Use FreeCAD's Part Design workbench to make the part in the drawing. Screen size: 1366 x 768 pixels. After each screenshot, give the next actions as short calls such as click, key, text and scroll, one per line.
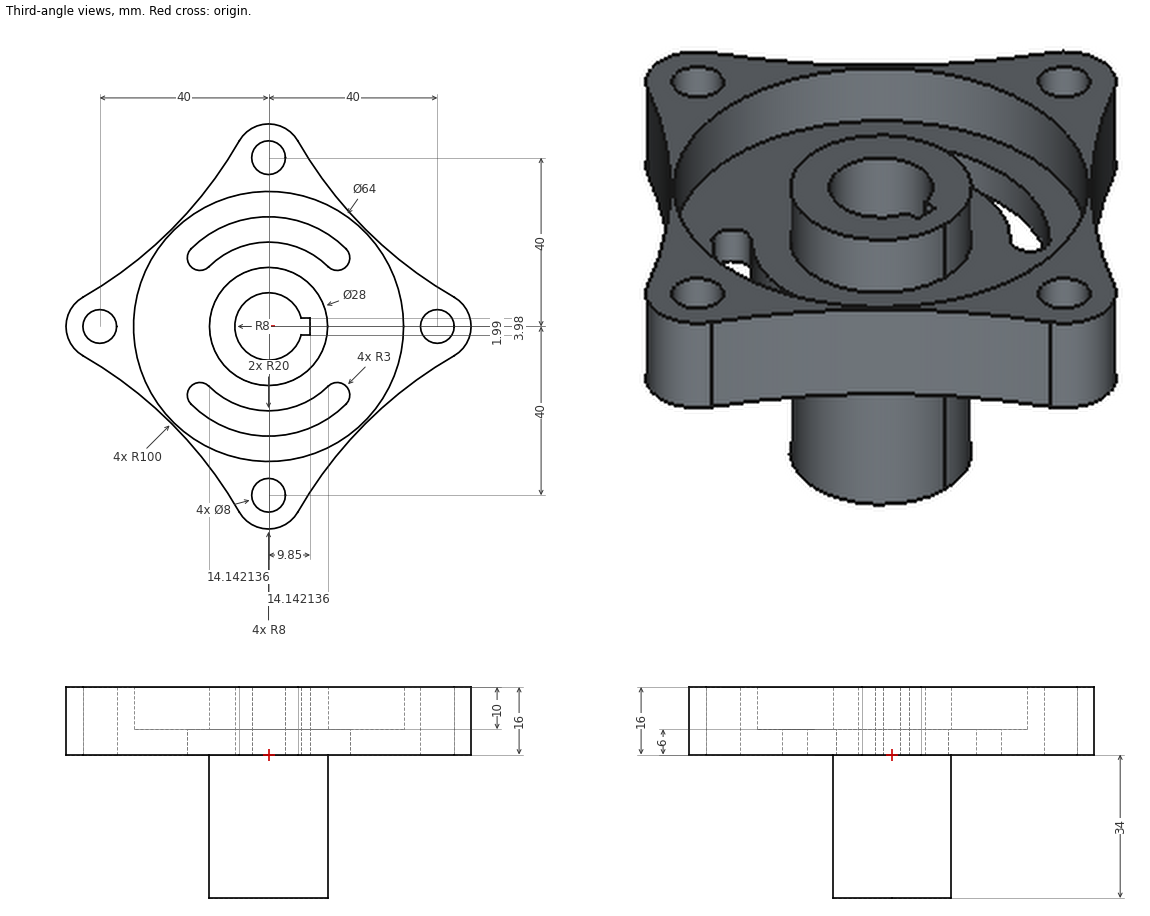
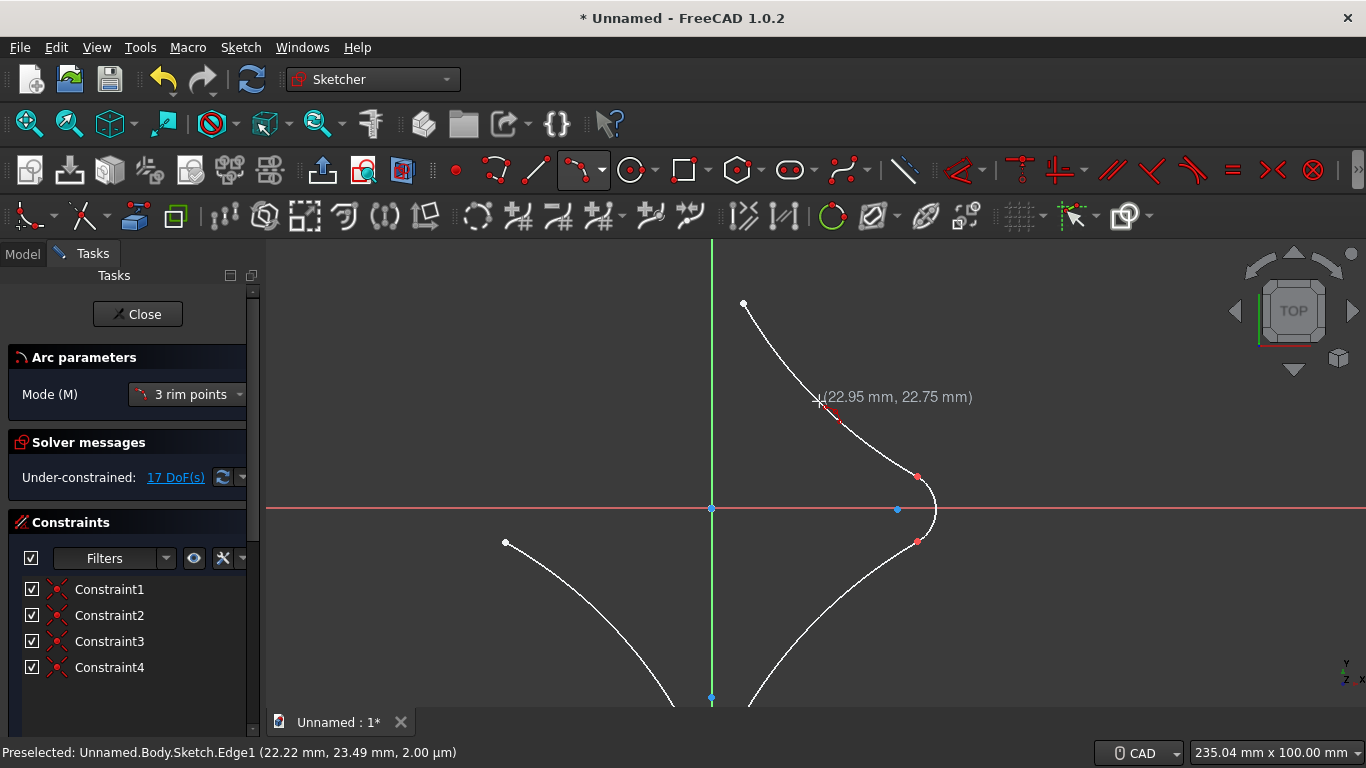
click(744, 304)
click(679, 303)
click(727, 287)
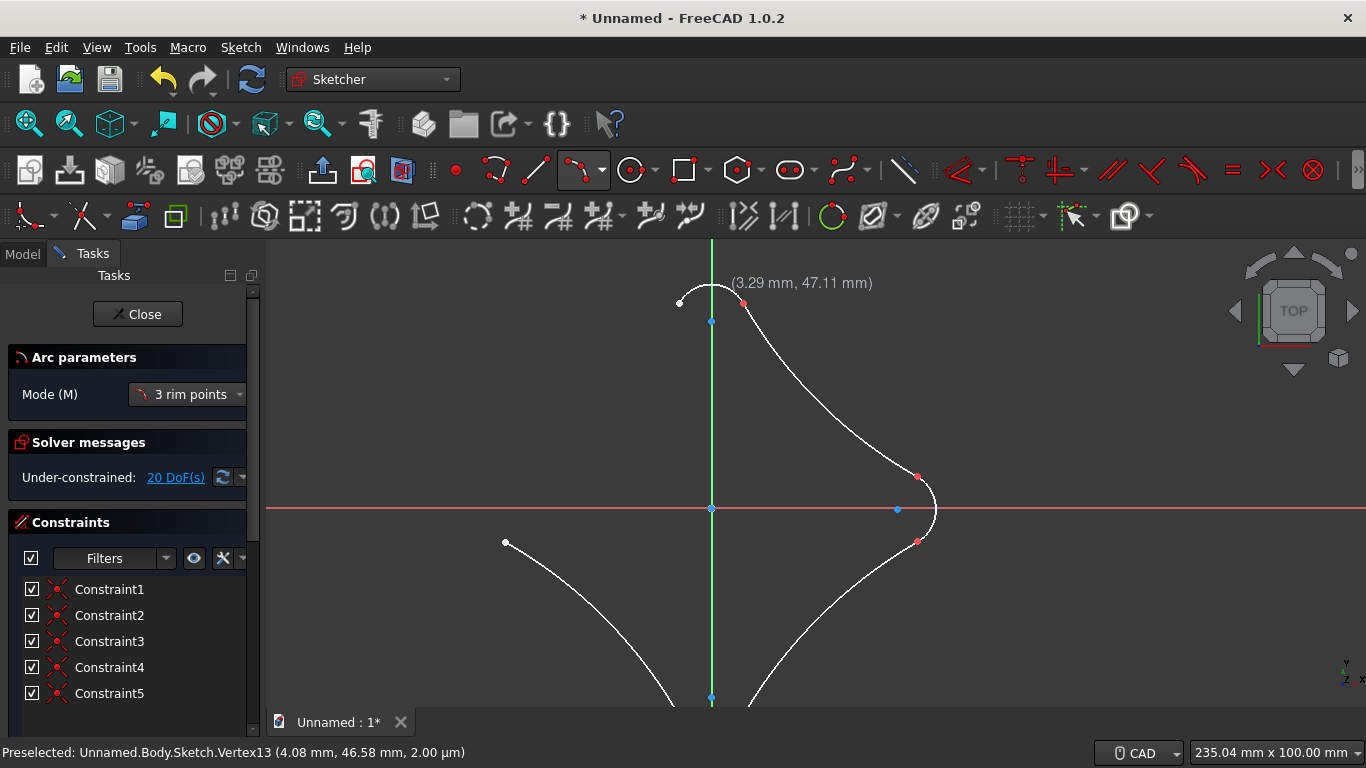
click(679, 304)
click(506, 476)
click(604, 401)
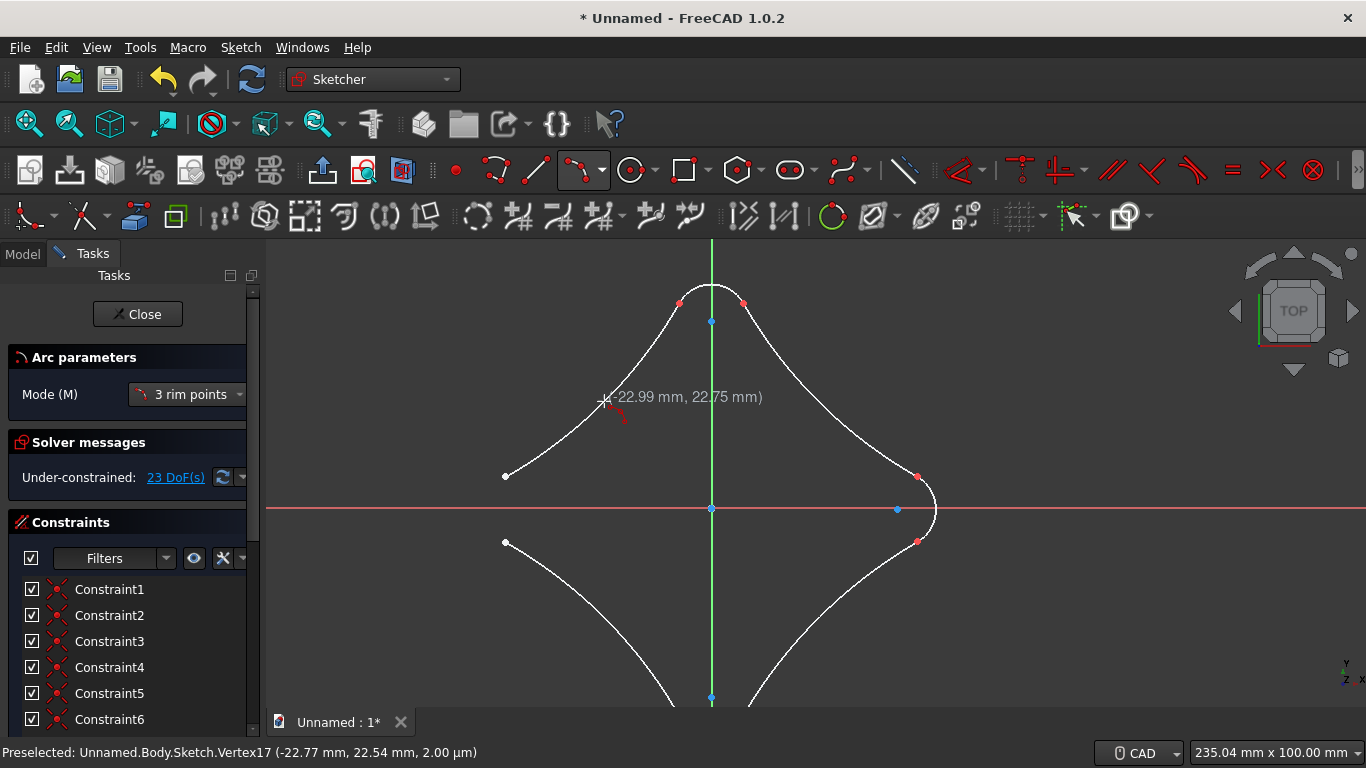
click(506, 477)
click(506, 543)
click(490, 493)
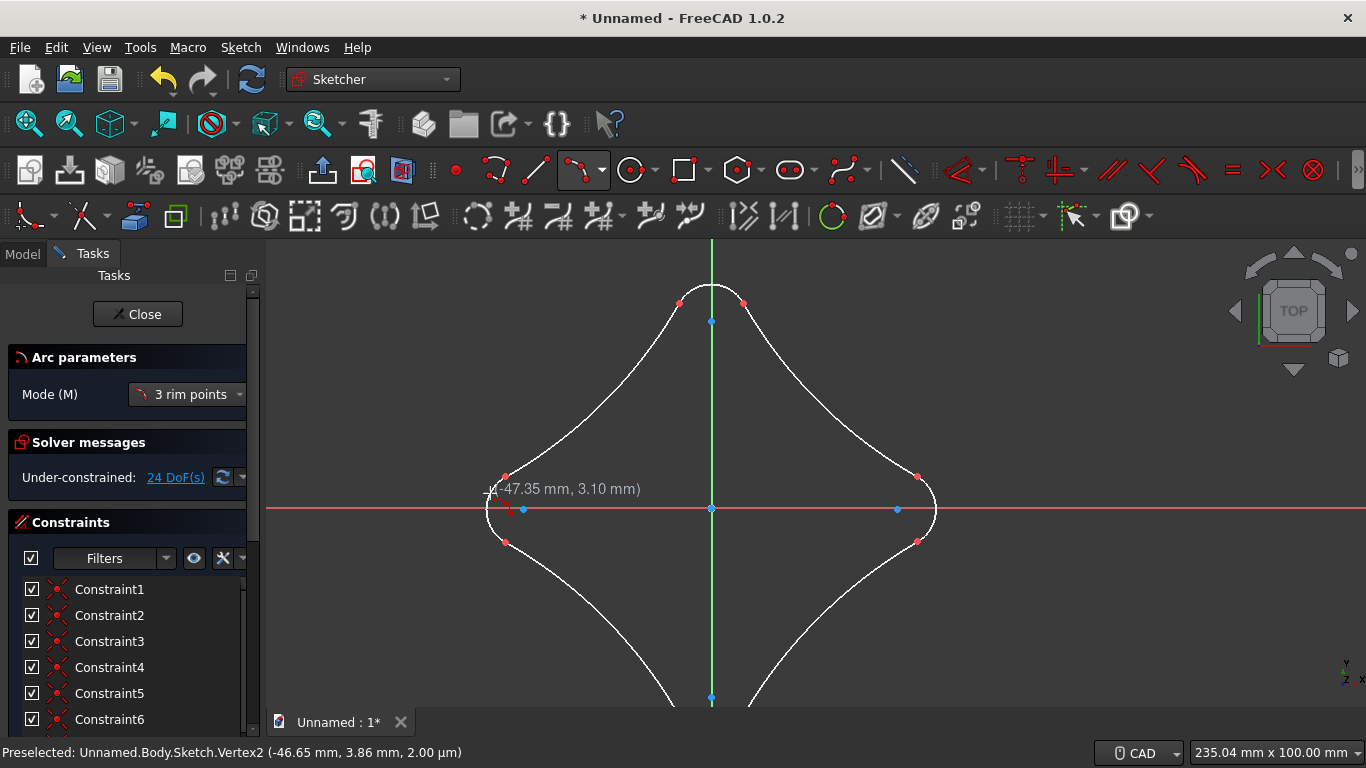
key(g)
key(c)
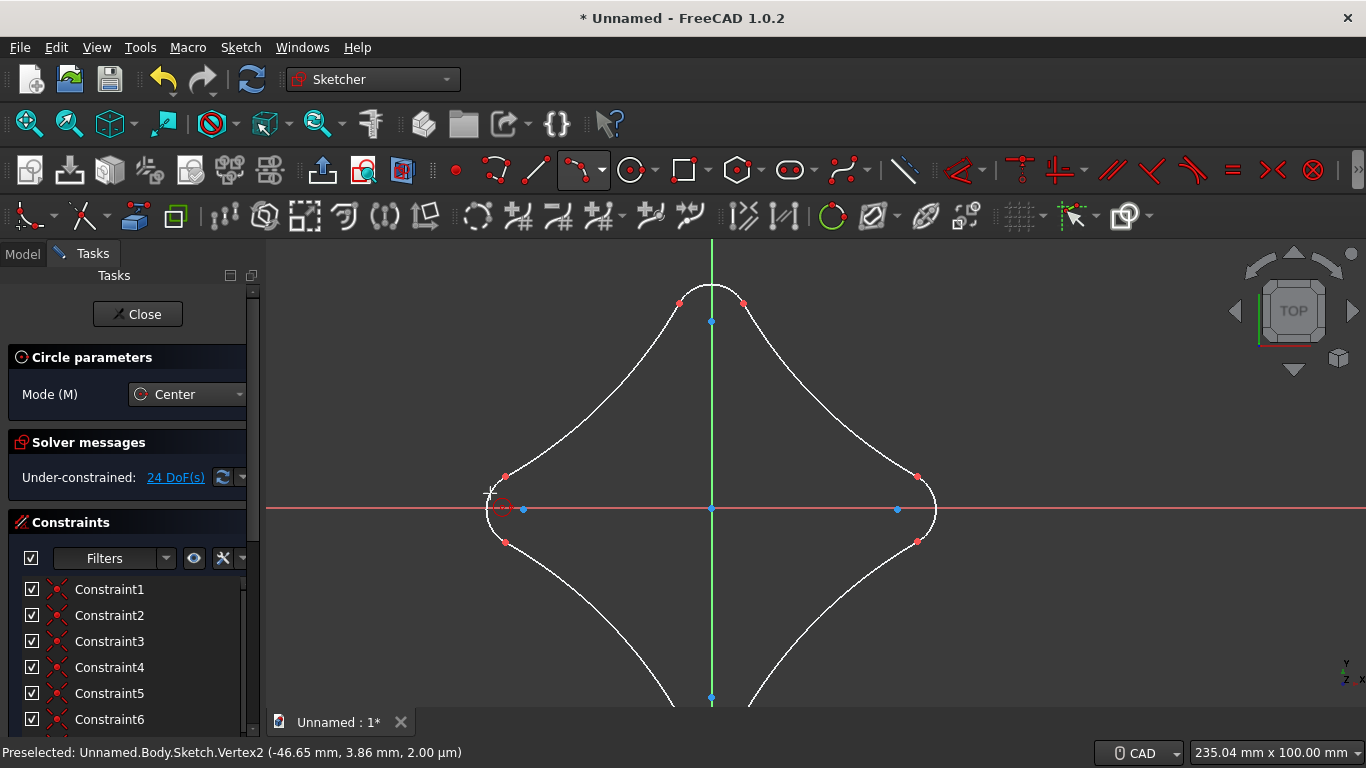
scroll(821, 401, down, 2)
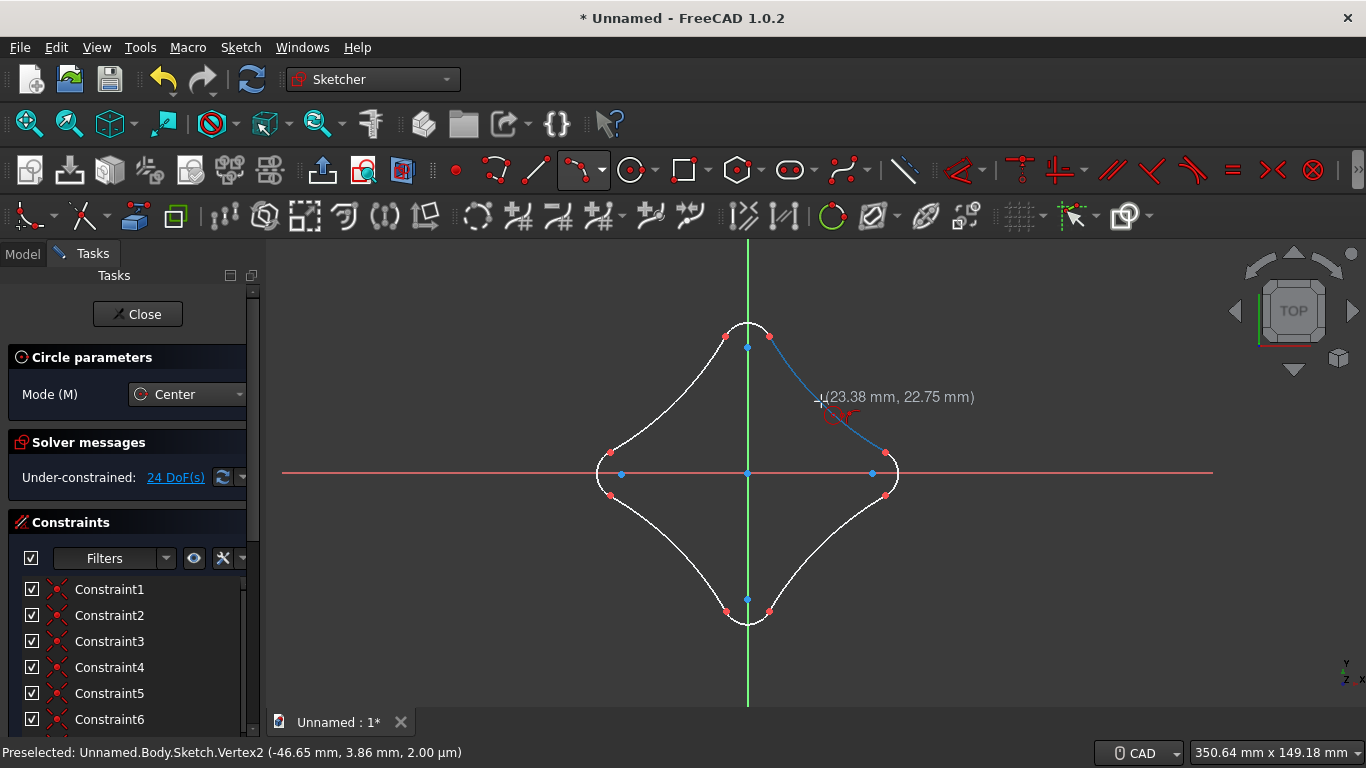
scroll(748, 599, up, 3)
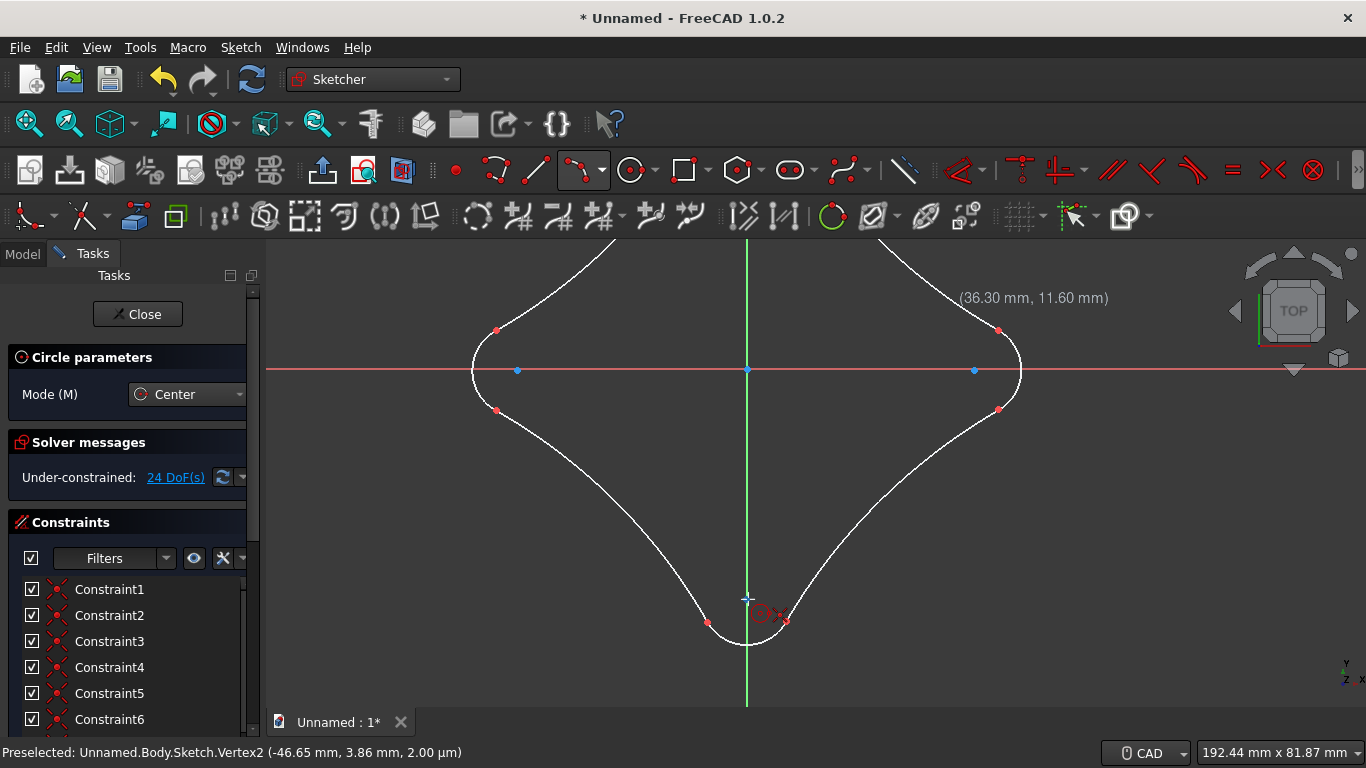
click(747, 598)
move(763, 582)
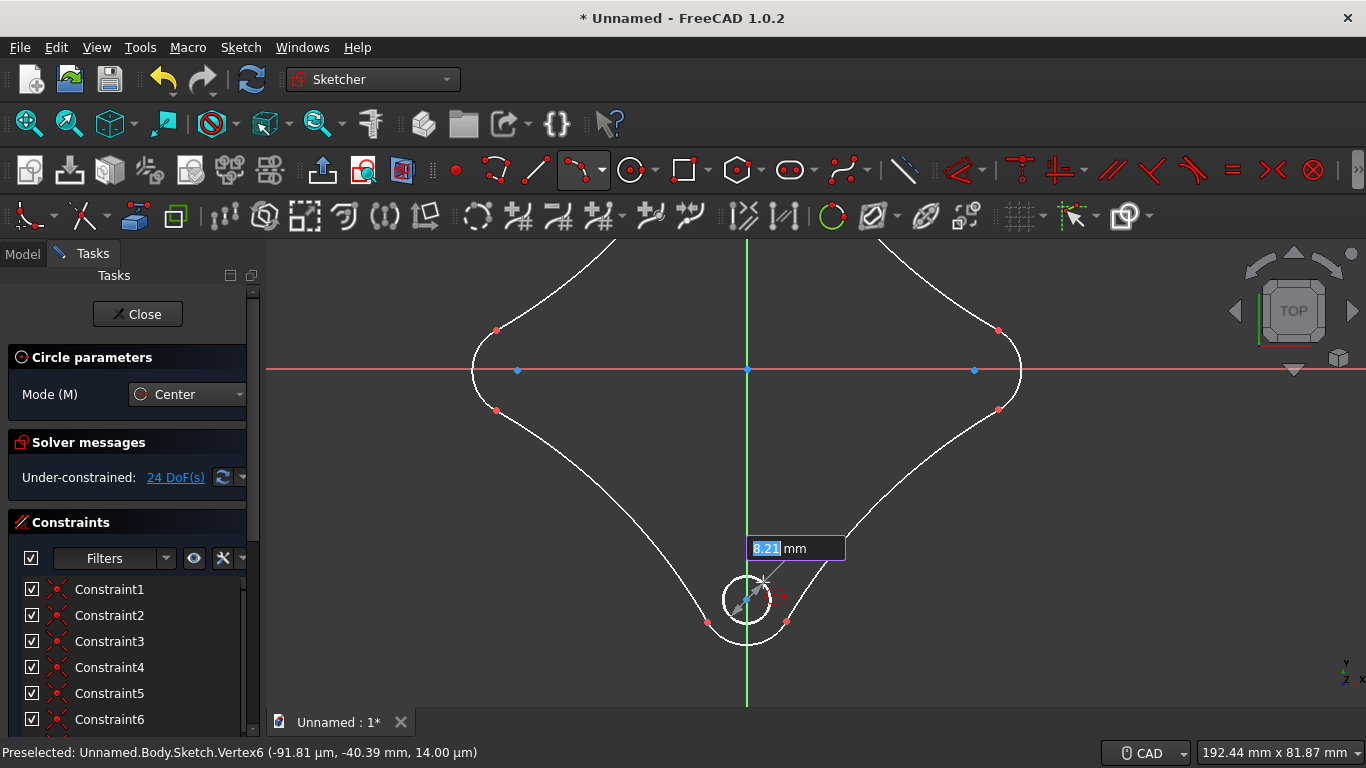
text(8)
key(Return)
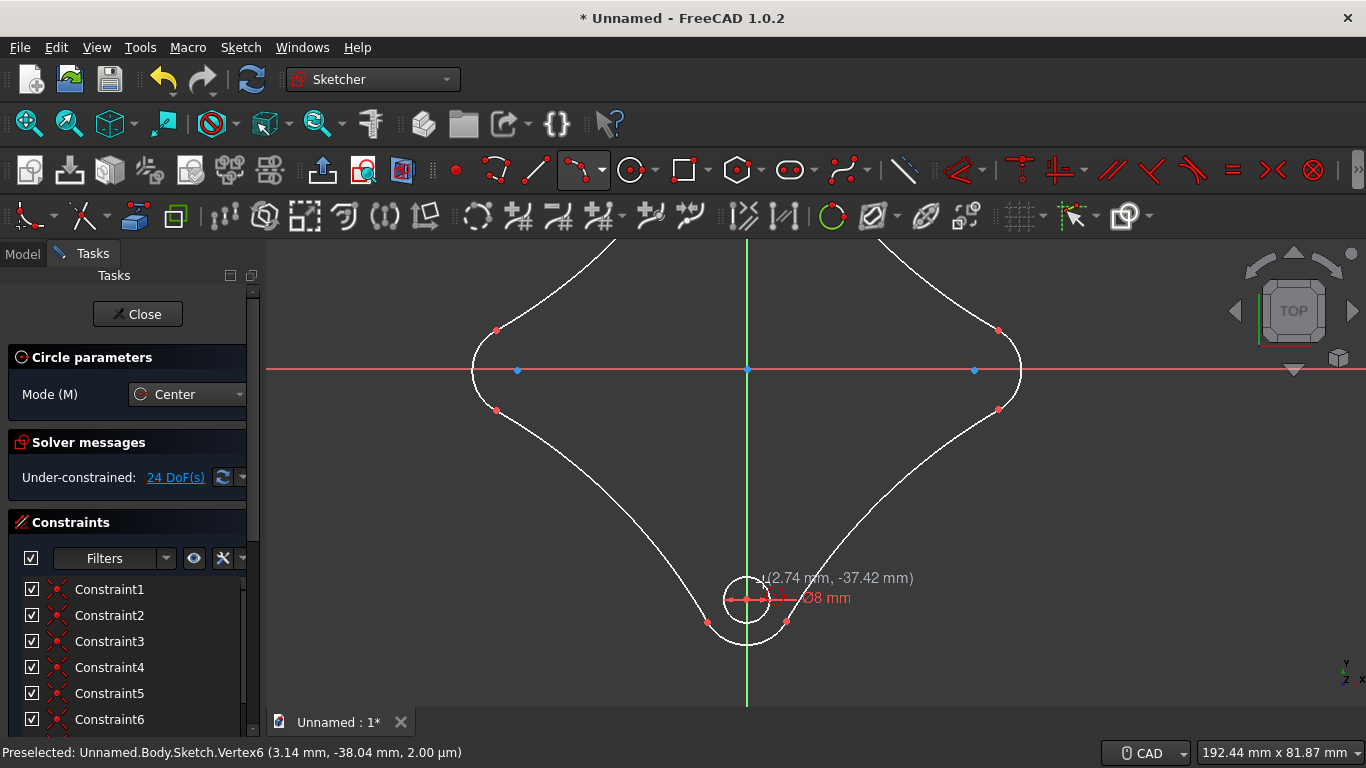
click(976, 369)
move(992, 353)